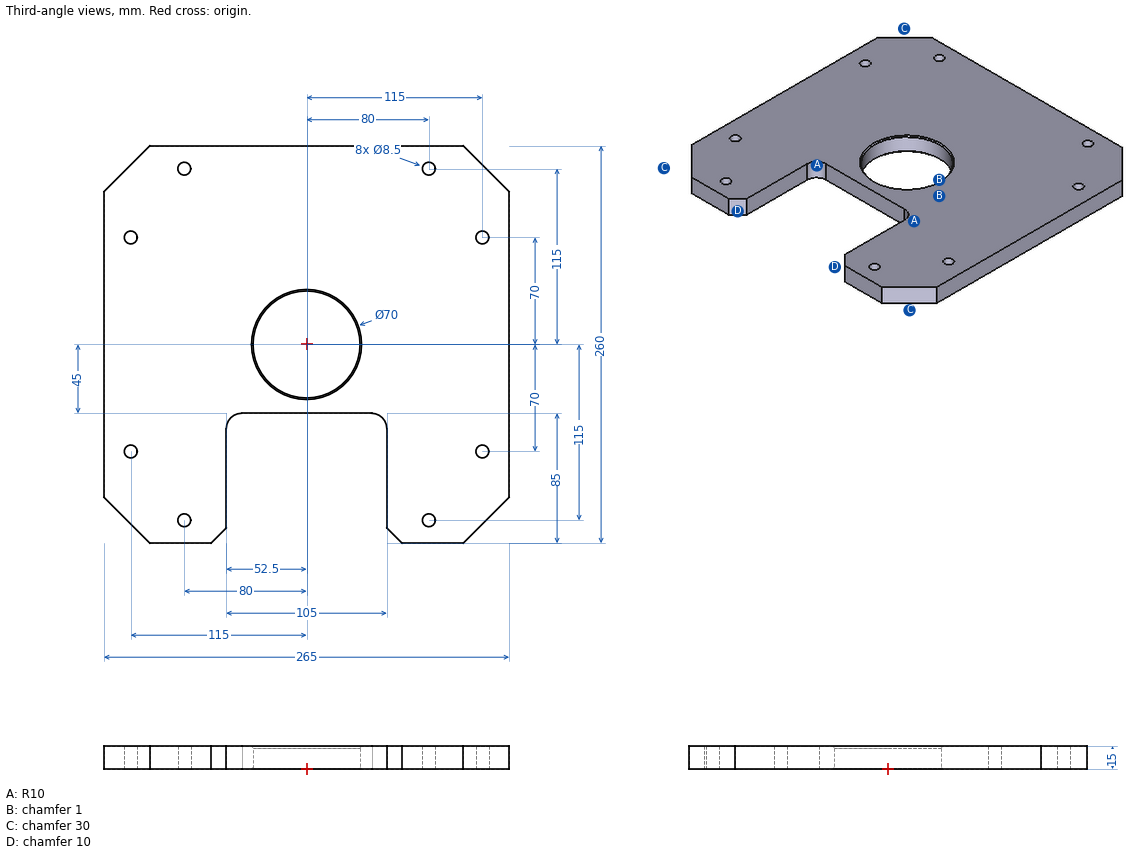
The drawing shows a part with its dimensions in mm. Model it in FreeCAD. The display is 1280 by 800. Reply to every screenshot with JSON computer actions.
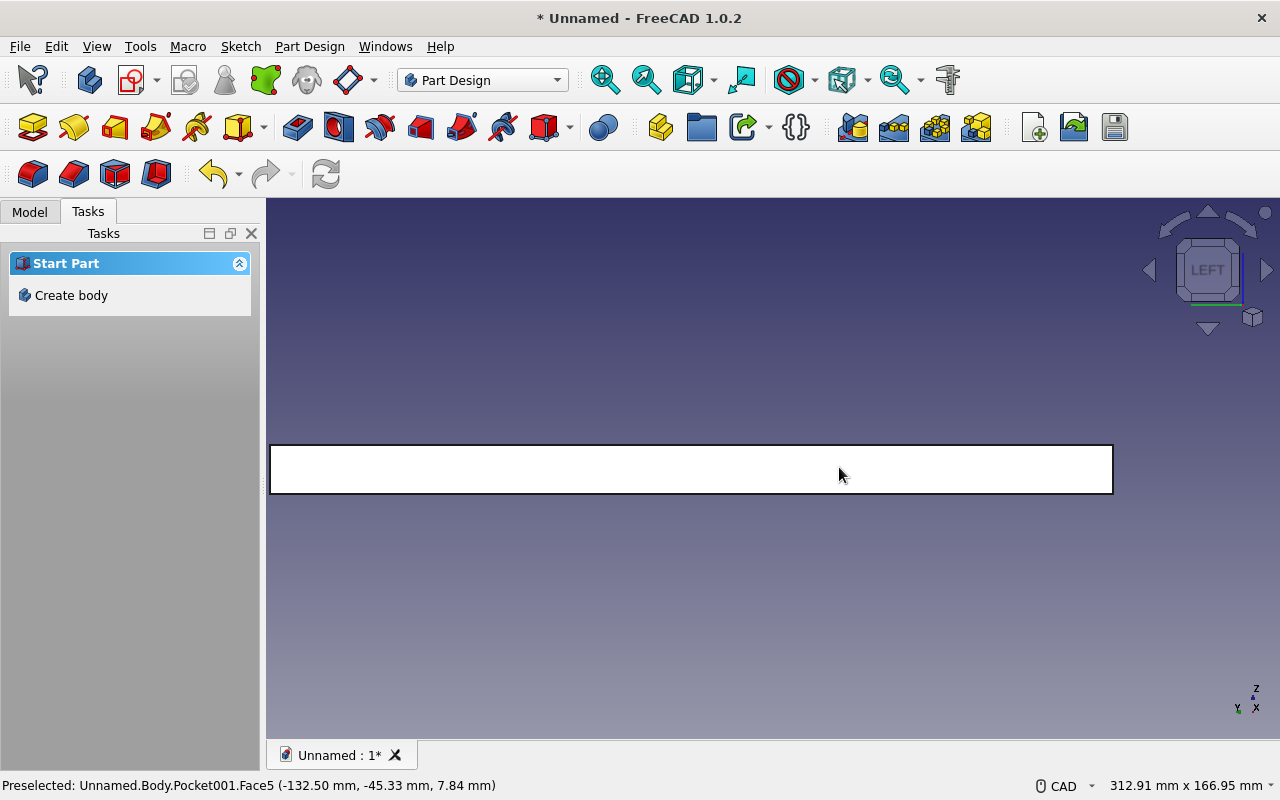
{"action": "left_click", "coordinate": [606, 80]}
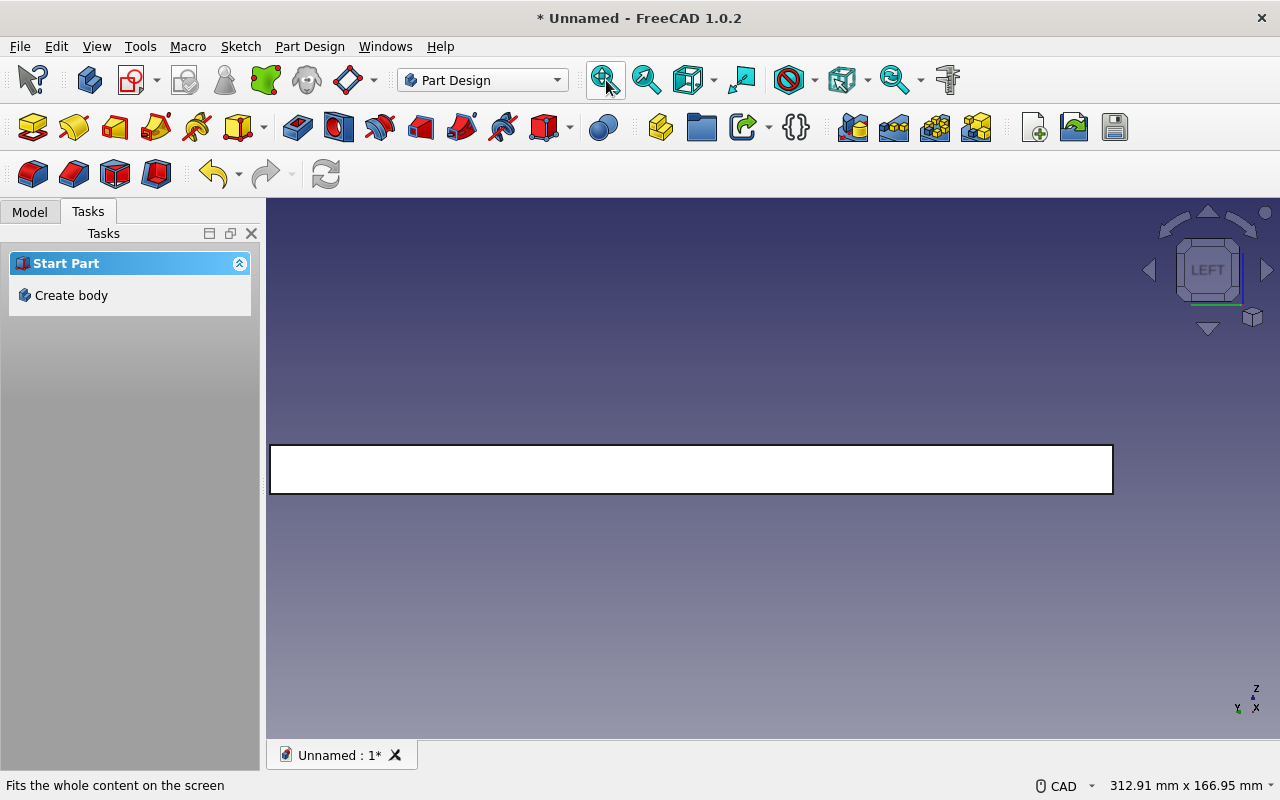
{"action": "key", "text": "v 3"}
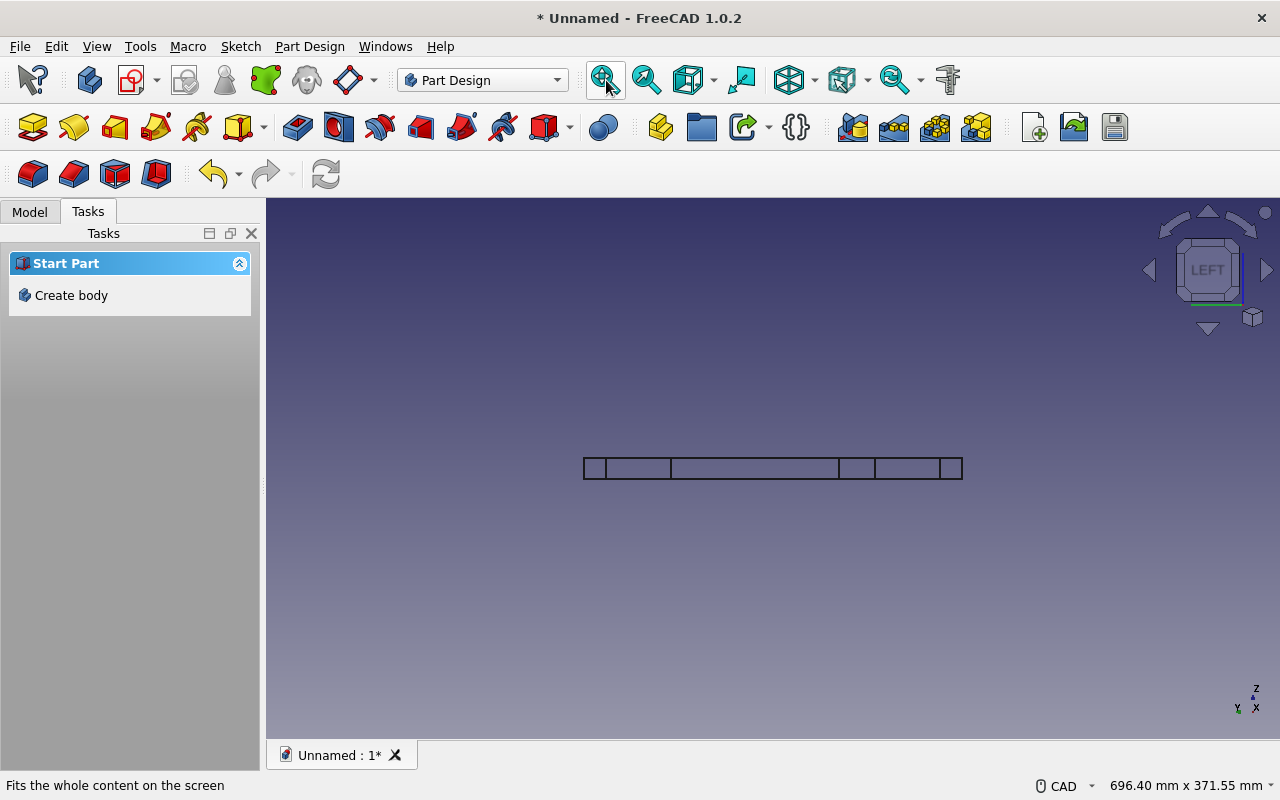
{"action": "key", "text": "0"}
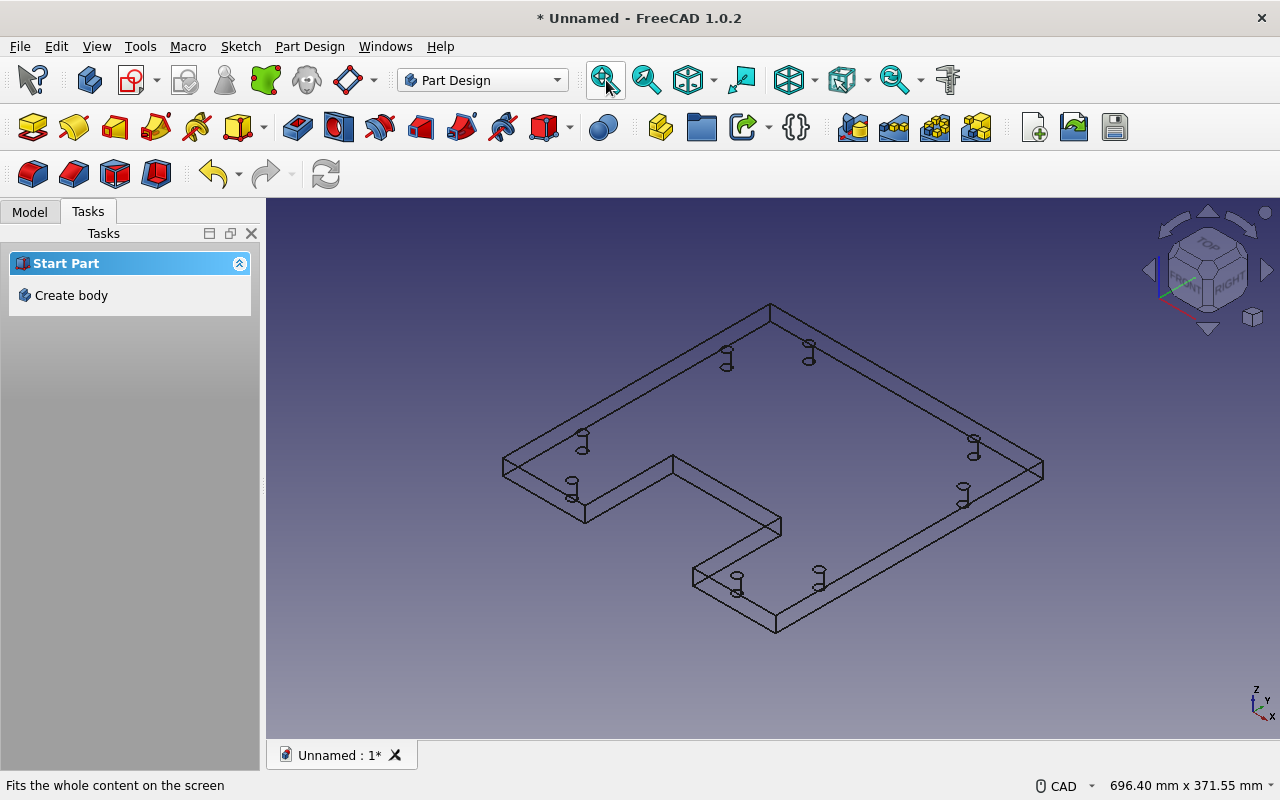
{"action": "left_click", "coordinate": [781, 525]}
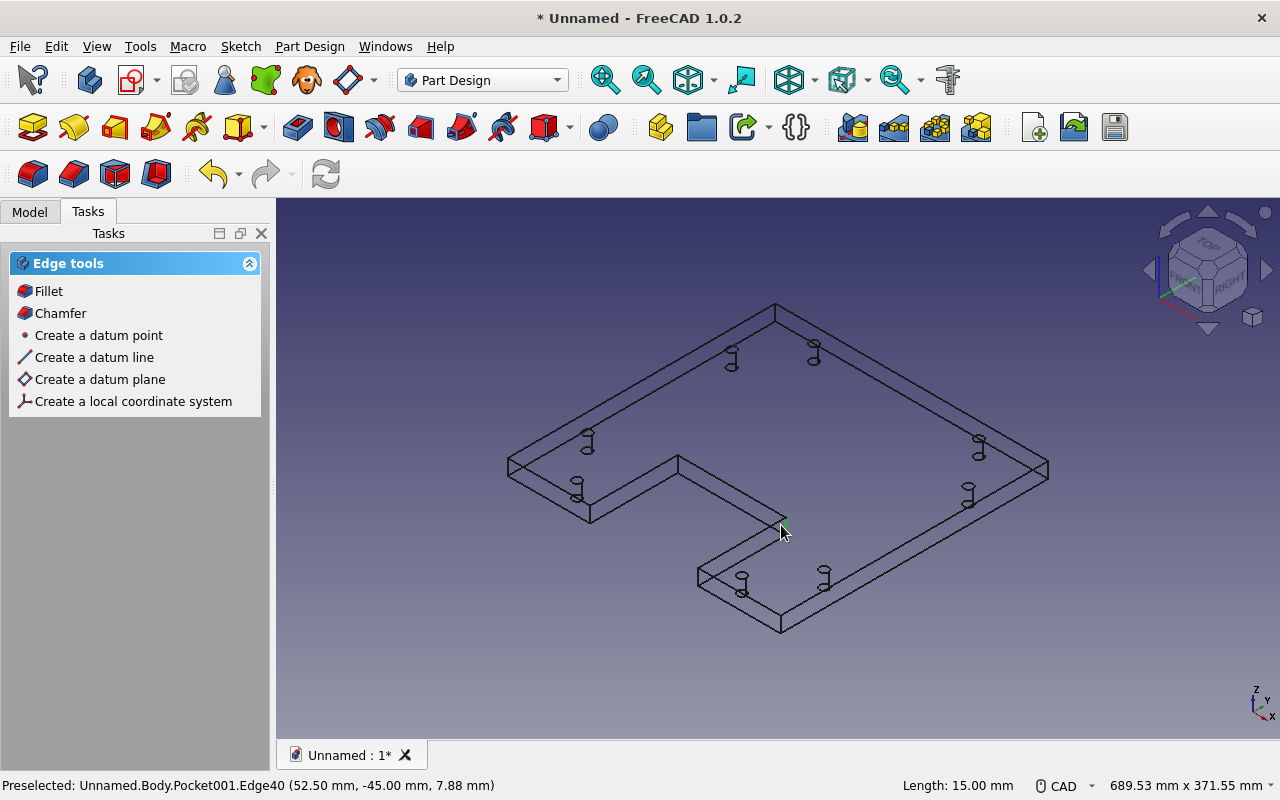
{"action": "left_click", "coordinate": [678, 463], "text": "ctrl"}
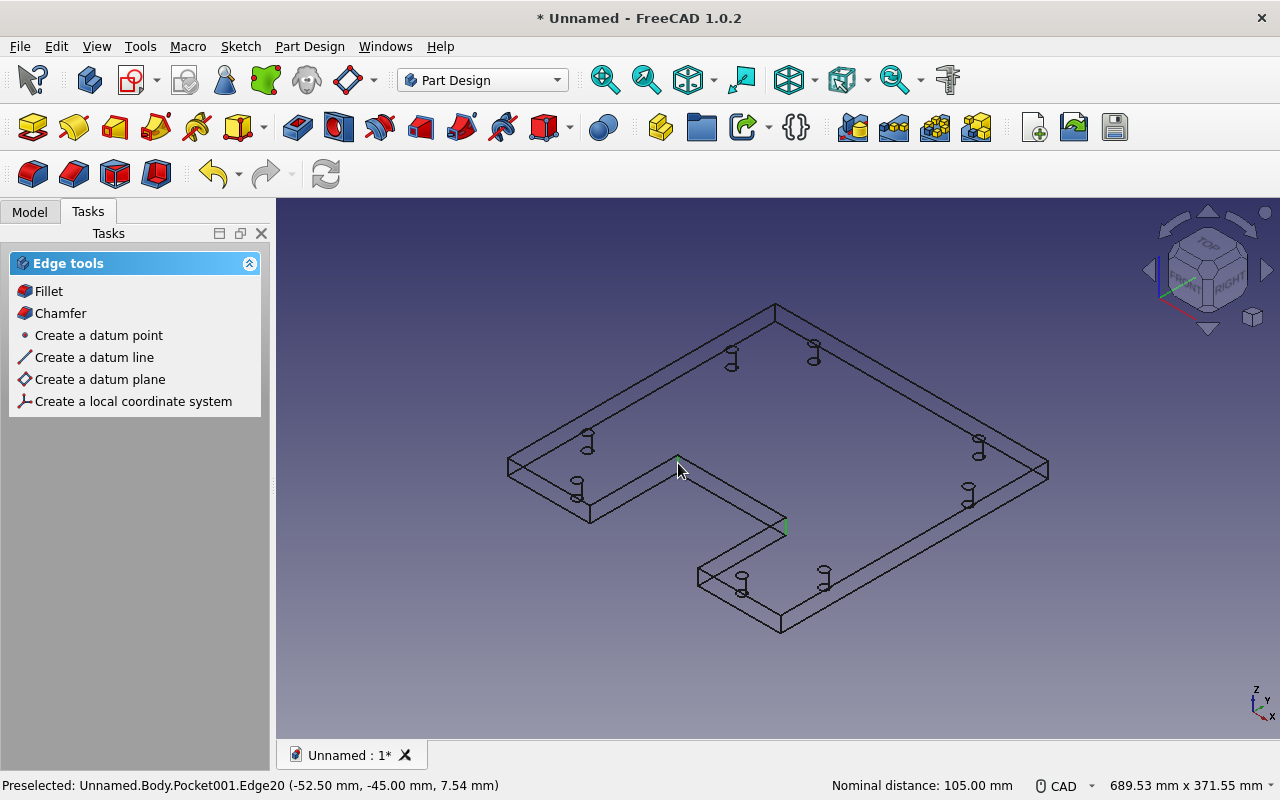
{"action": "key", "text": "v 1"}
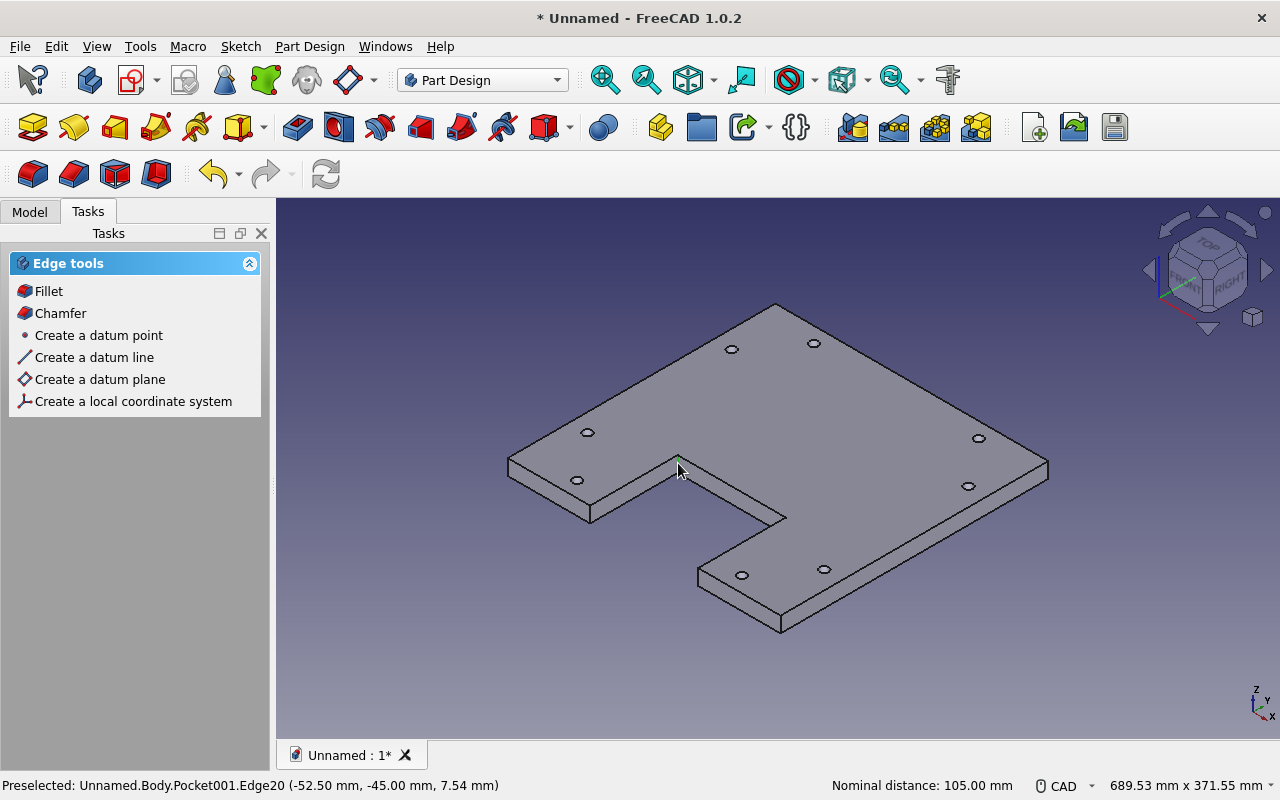
{"action": "left_click", "coordinate": [33, 174]}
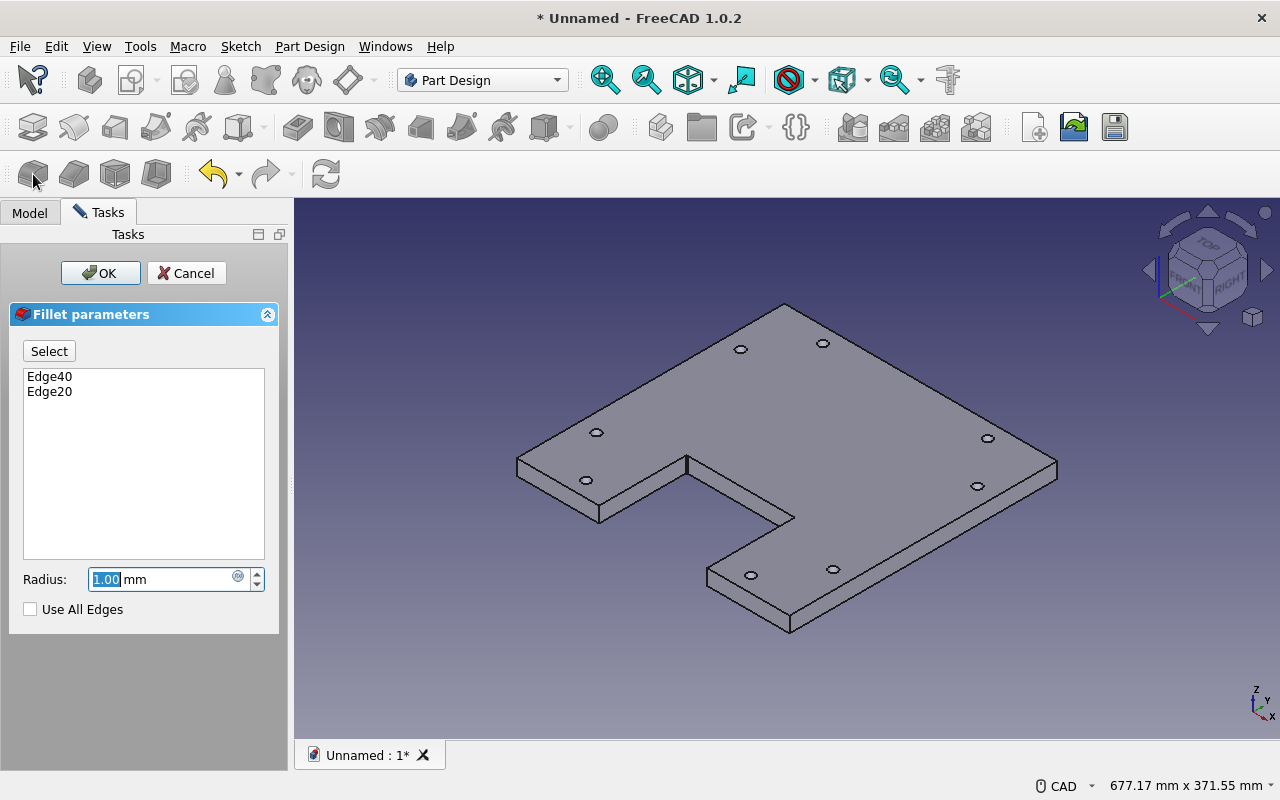
{"action": "type", "text": "10"}
{"action": "key", "text": "Tab"}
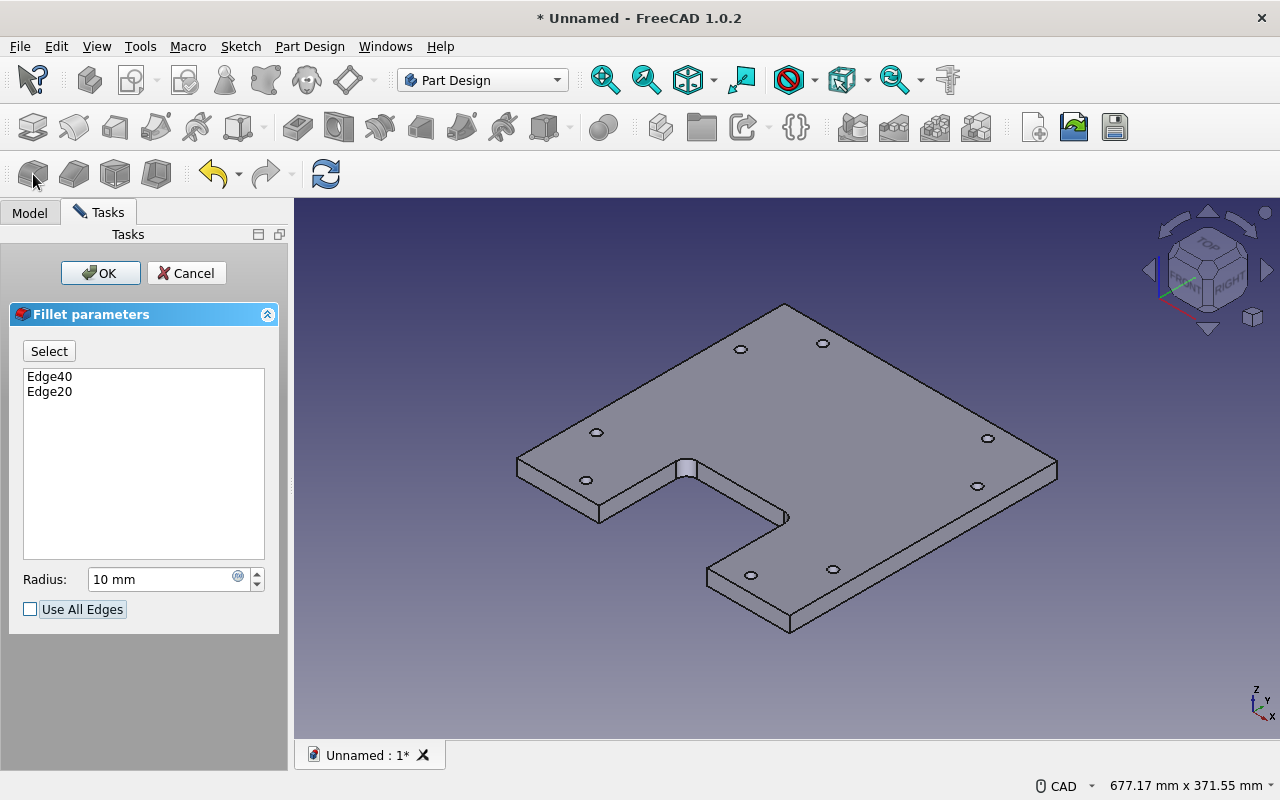
{"action": "left_click", "coordinate": [101, 273]}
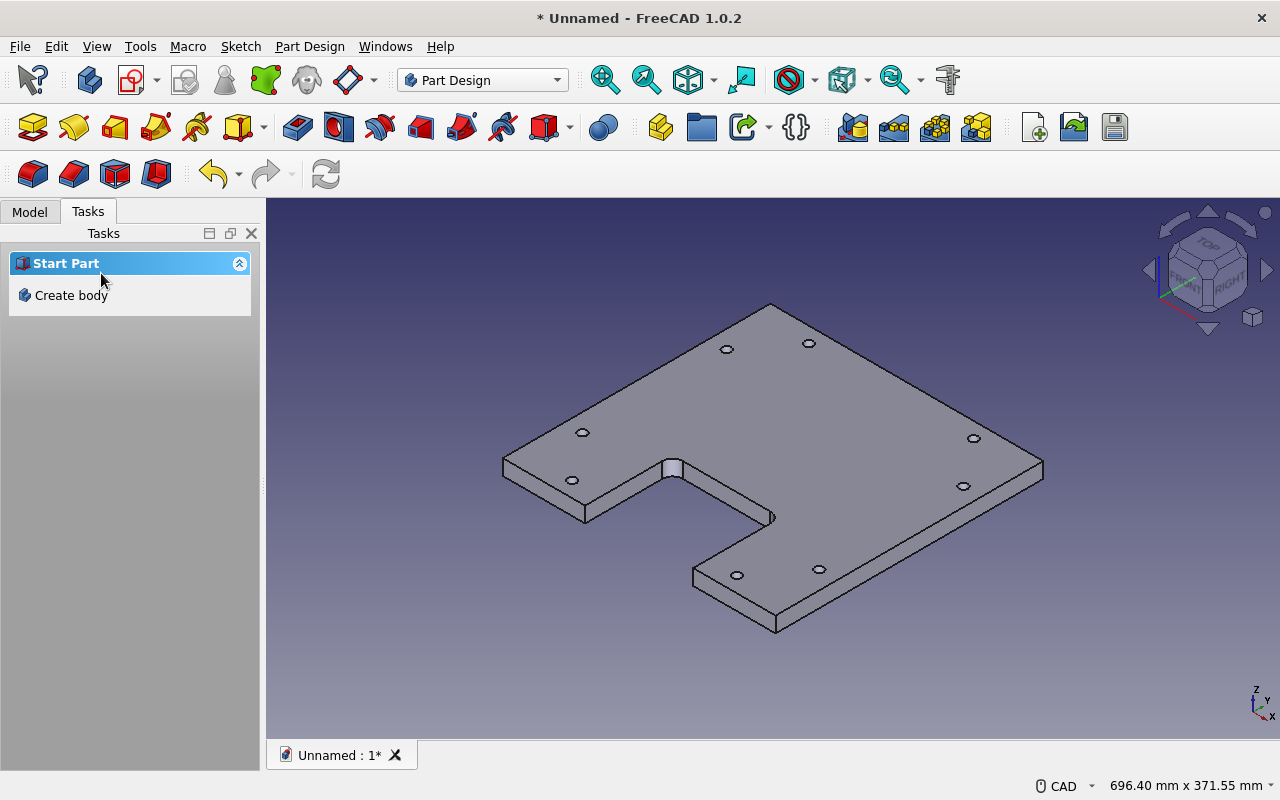
{"action": "left_click", "coordinate": [130, 80]}